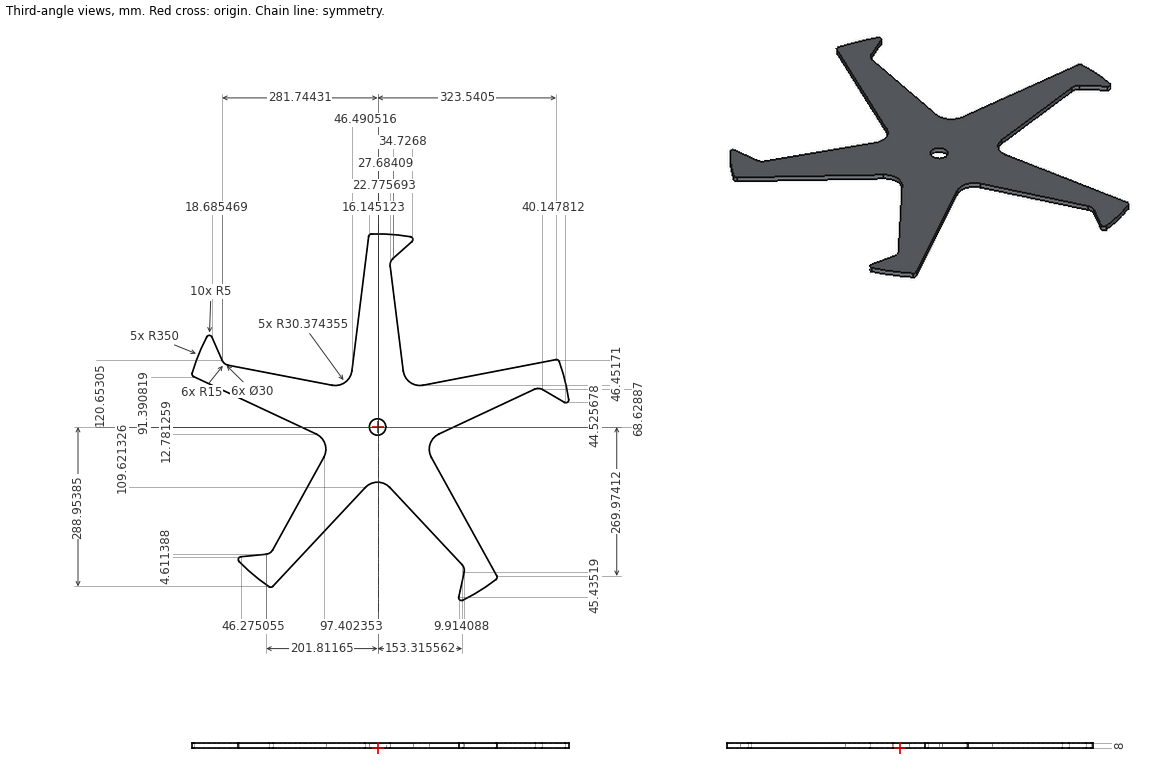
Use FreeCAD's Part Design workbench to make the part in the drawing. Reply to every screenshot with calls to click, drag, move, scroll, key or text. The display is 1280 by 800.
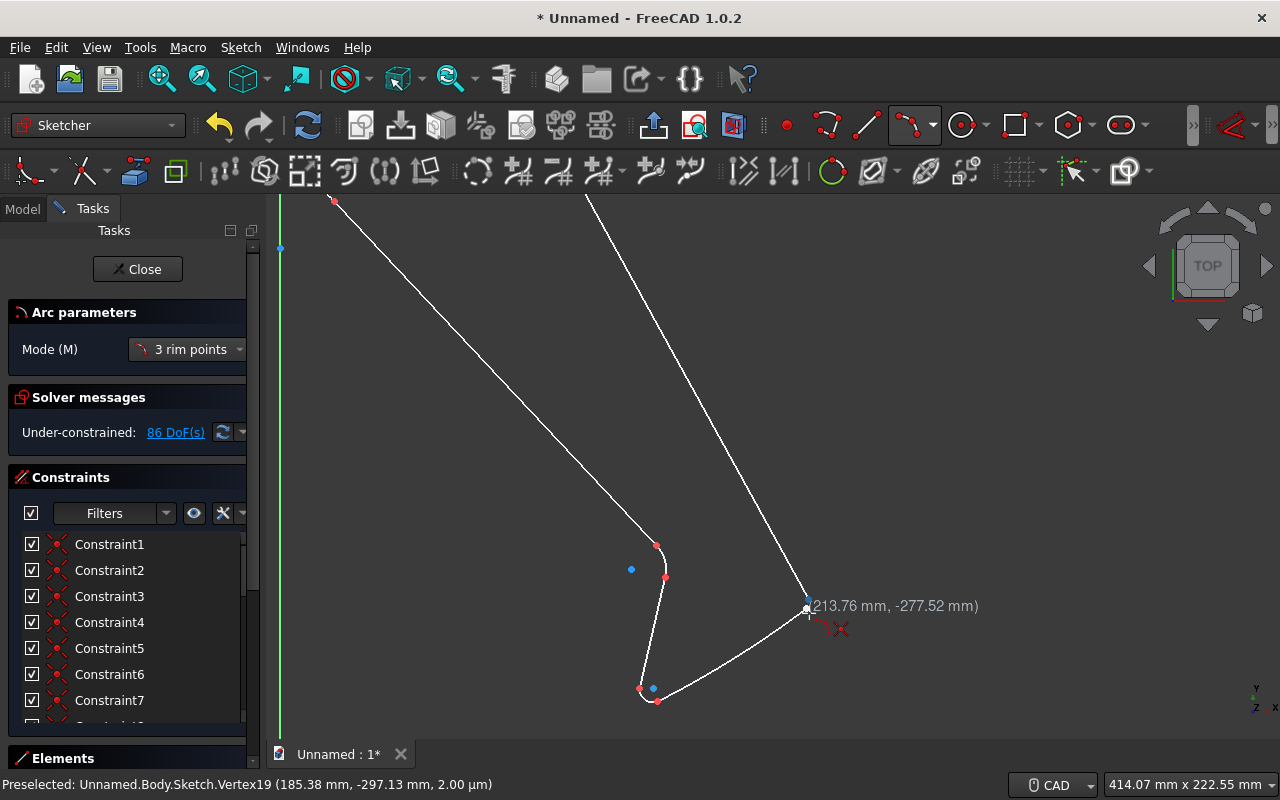
click(807, 609)
click(809, 599)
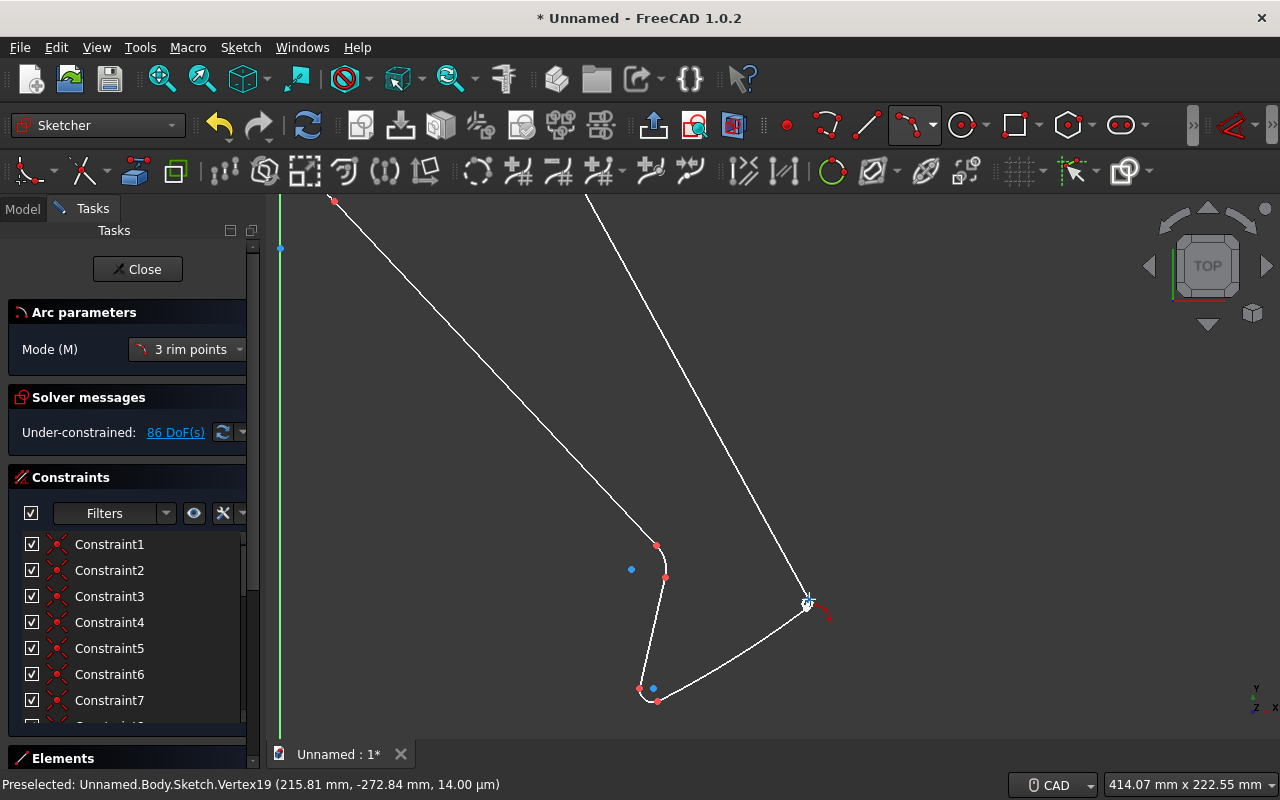
scroll(811, 601, up, 9)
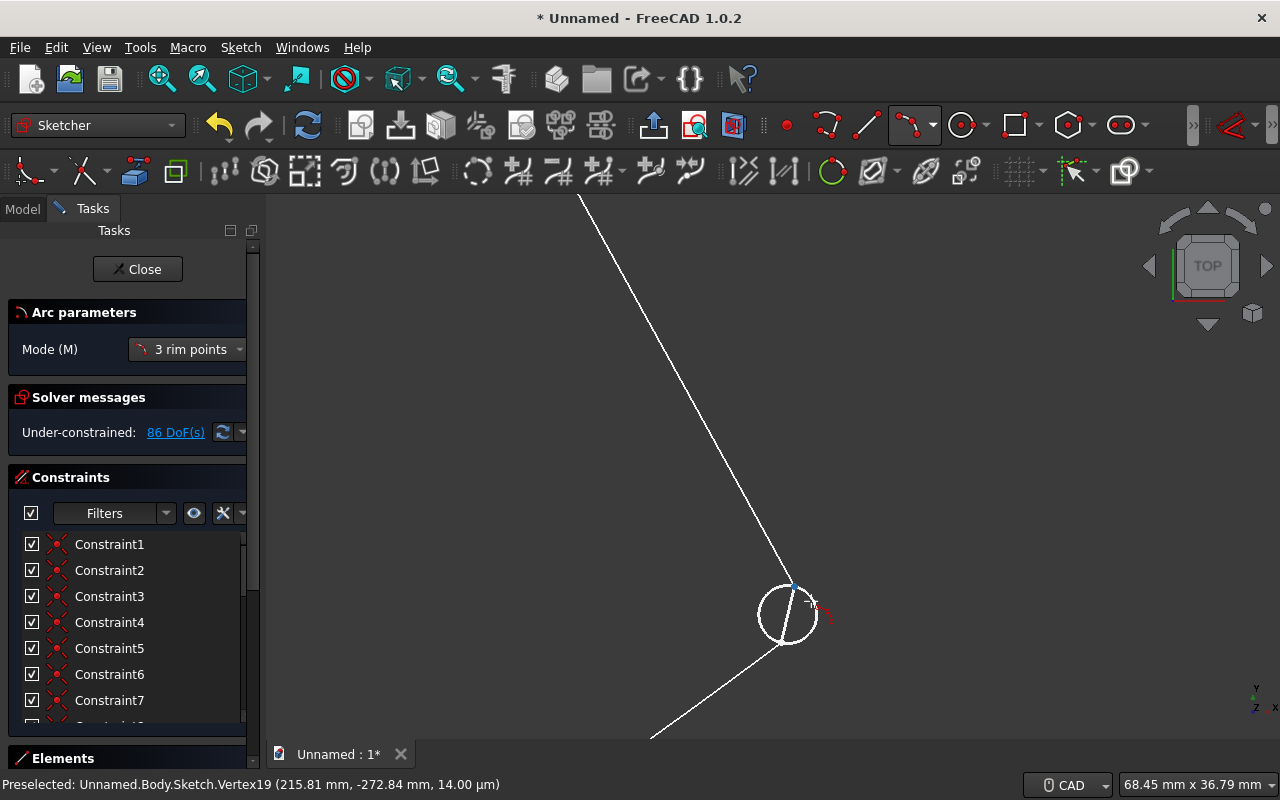
click(807, 595)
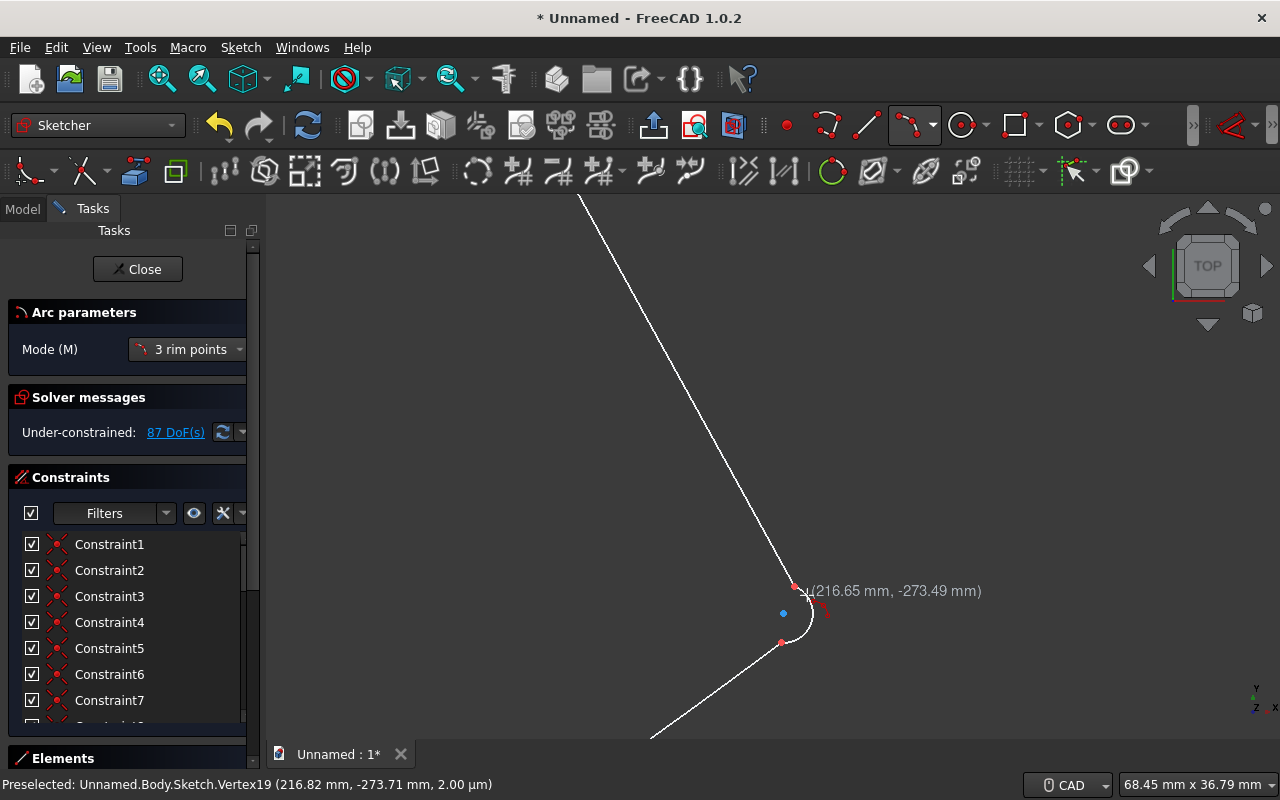
scroll(833, 644, down, 16)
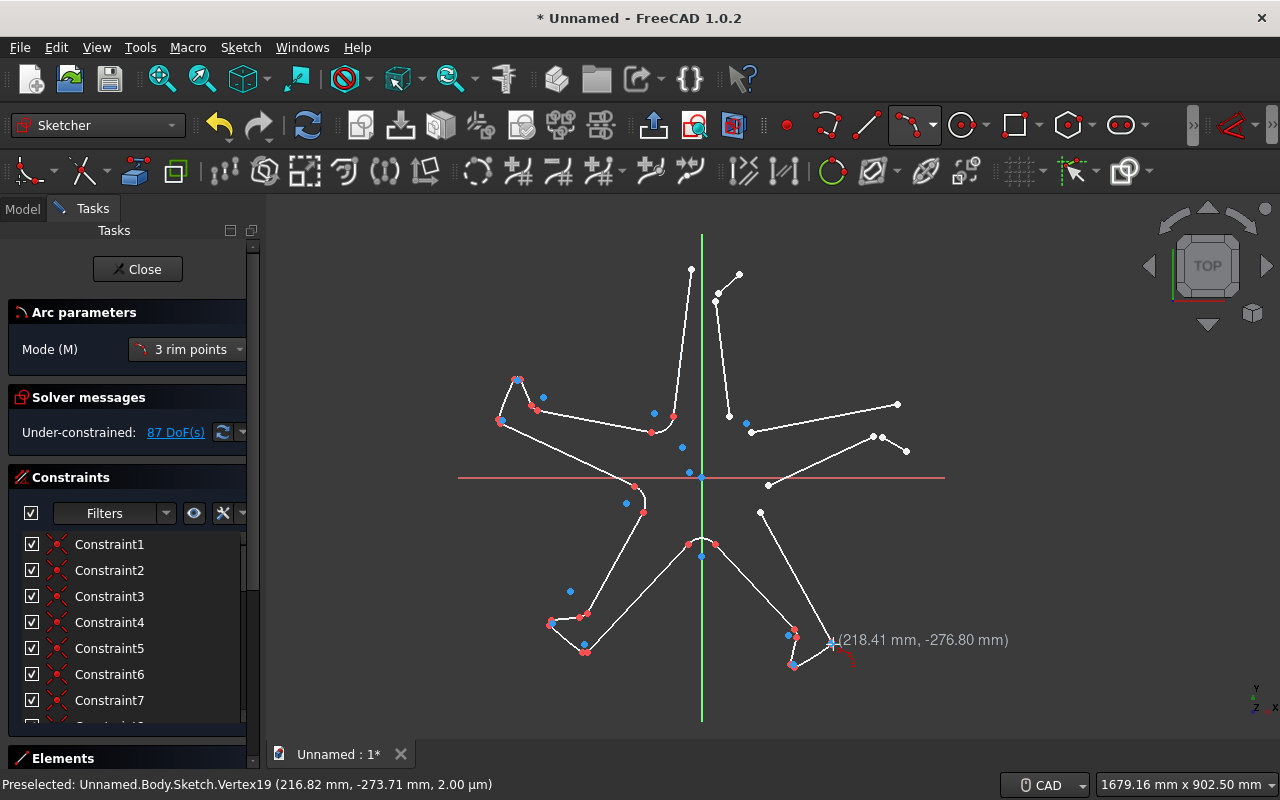
click(760, 512)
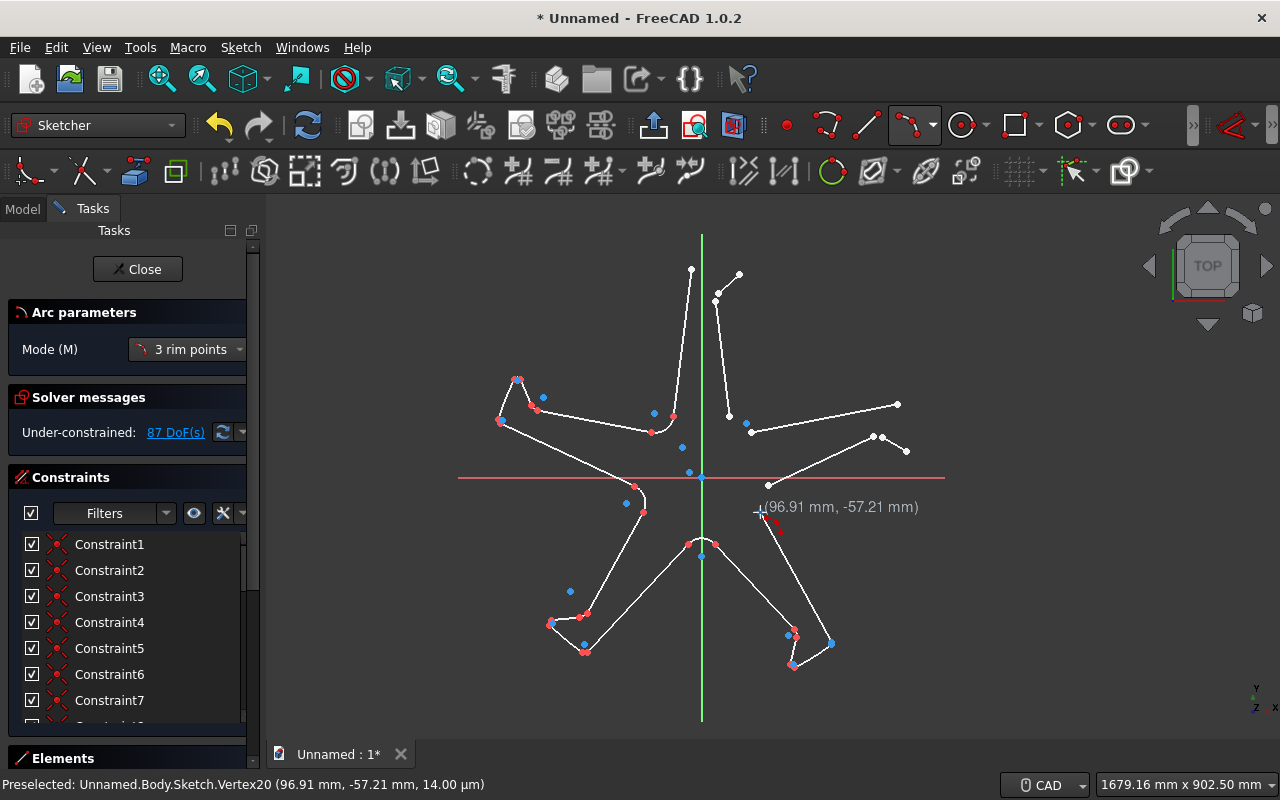
scroll(769, 485, up, 4)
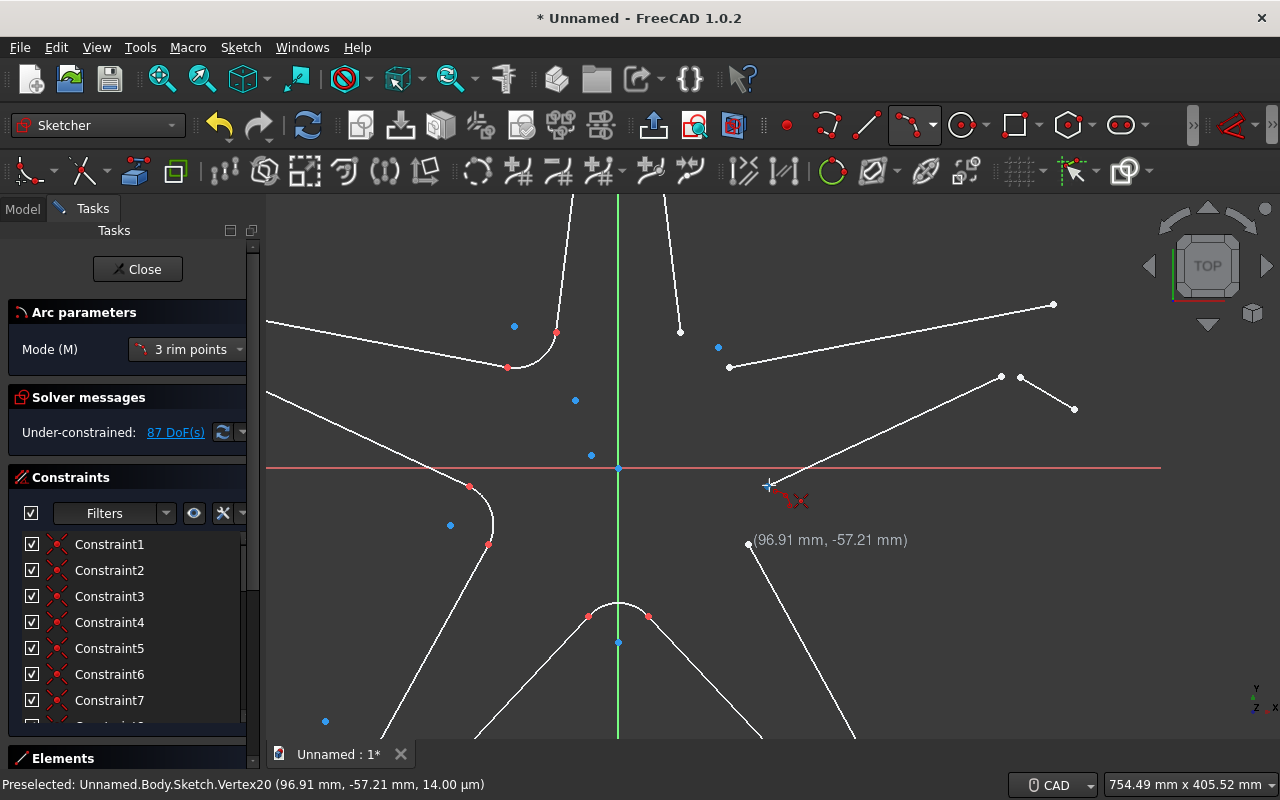
click(768, 486)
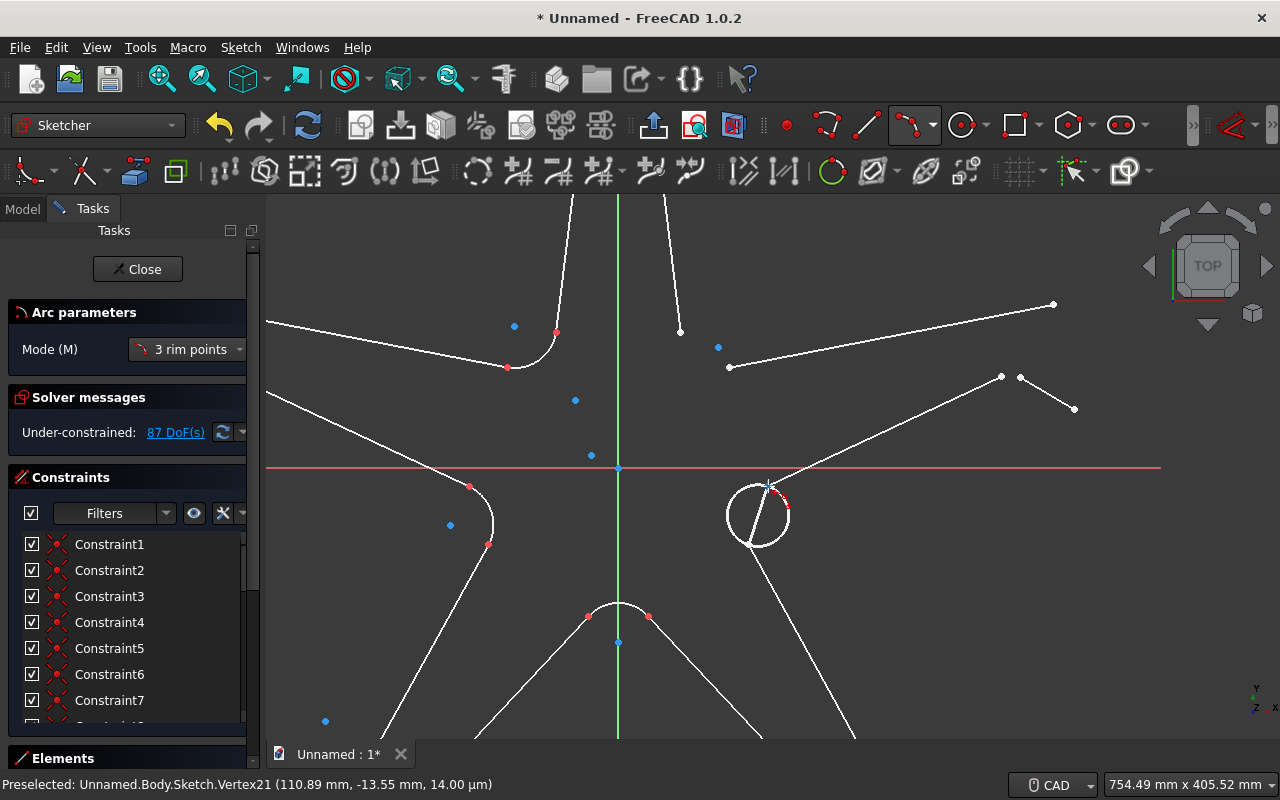
scroll(746, 510, up, 2)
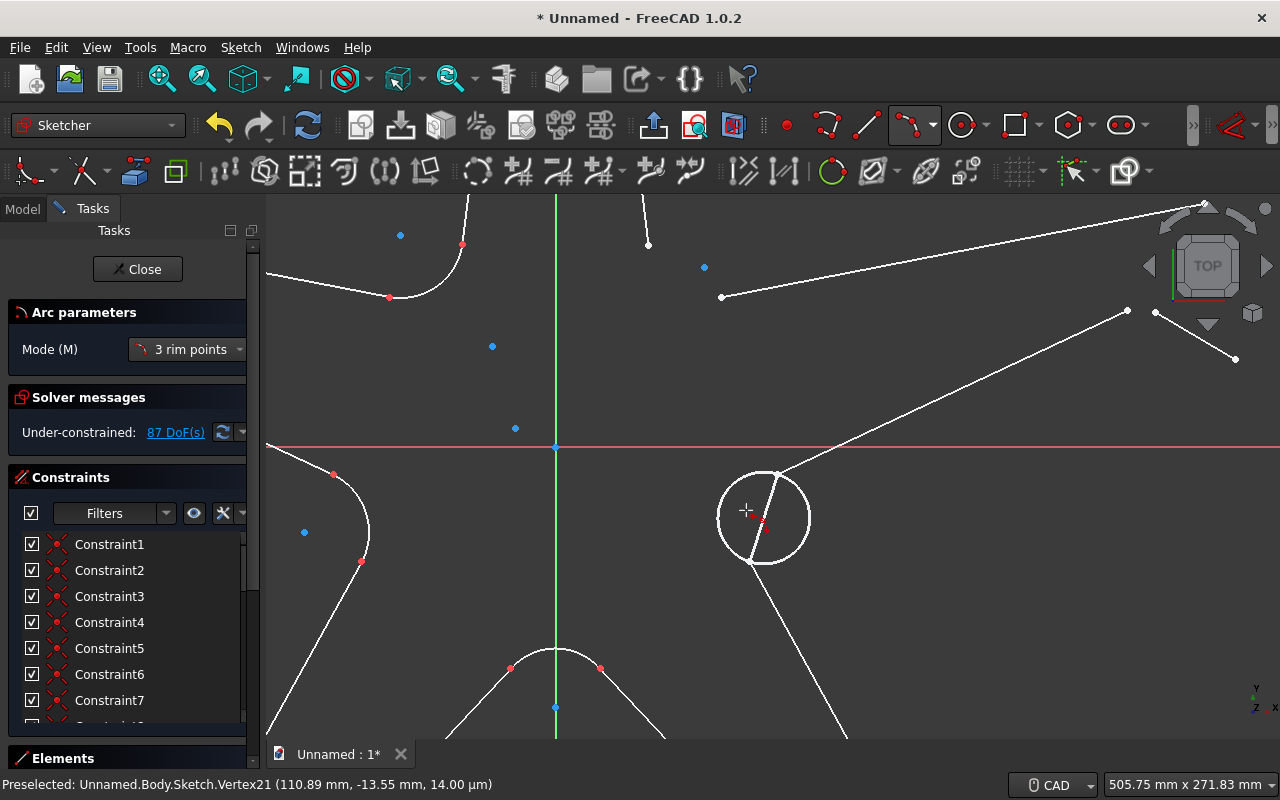
click(746, 509)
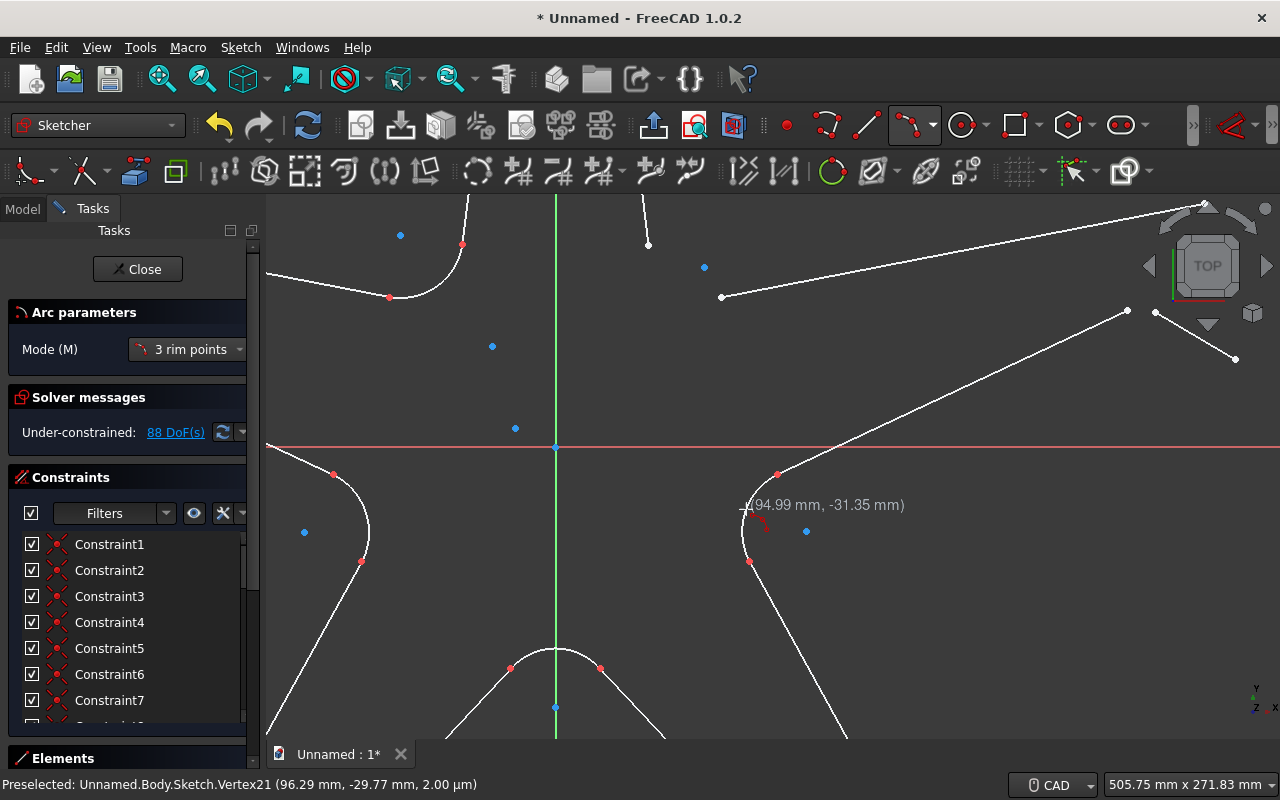
scroll(750, 485, down, 7)